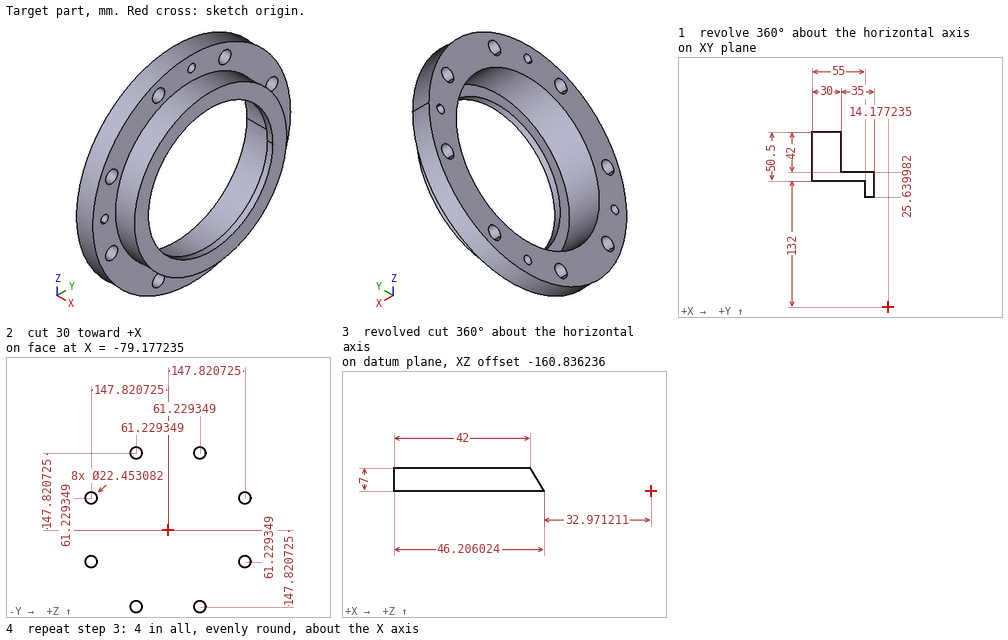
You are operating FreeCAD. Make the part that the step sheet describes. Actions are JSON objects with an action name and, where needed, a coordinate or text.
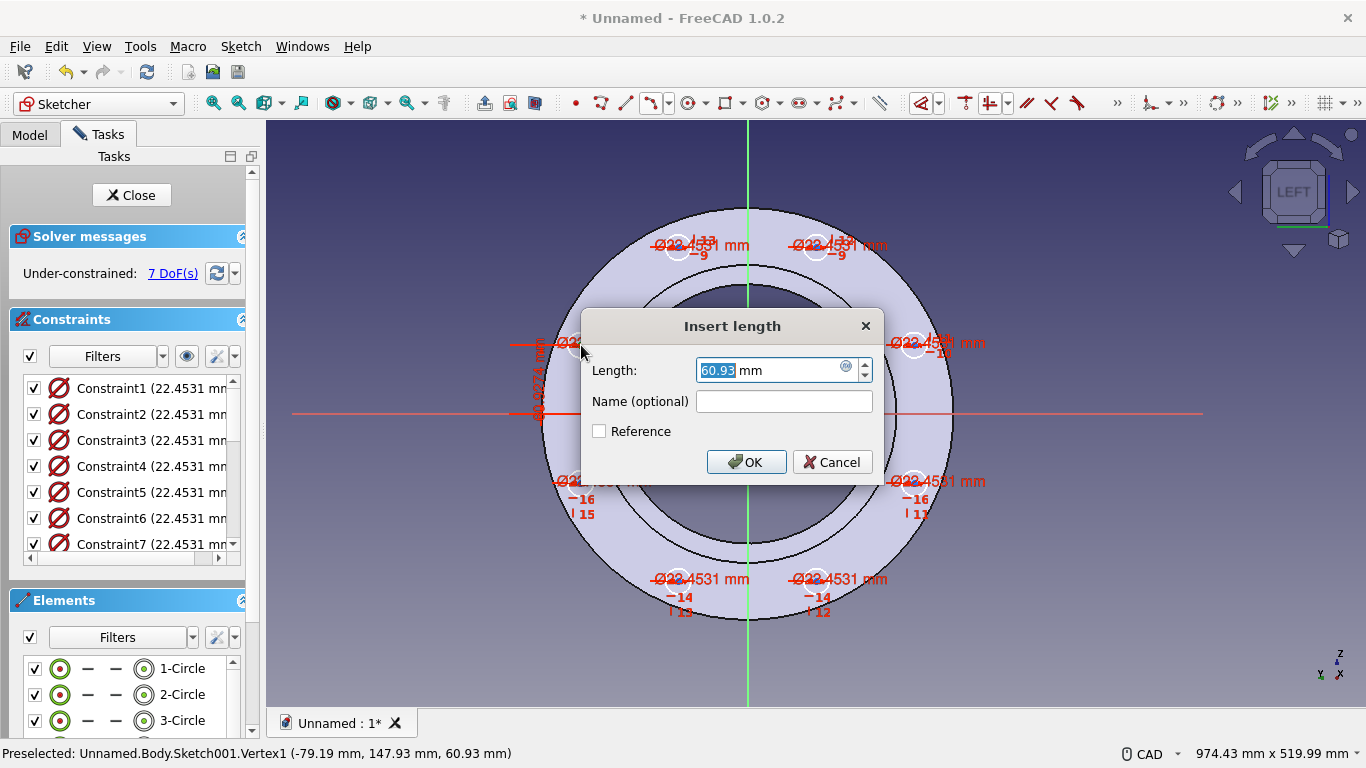
{"action": "type", "text": "61.229349"}
{"action": "key", "text": "Return"}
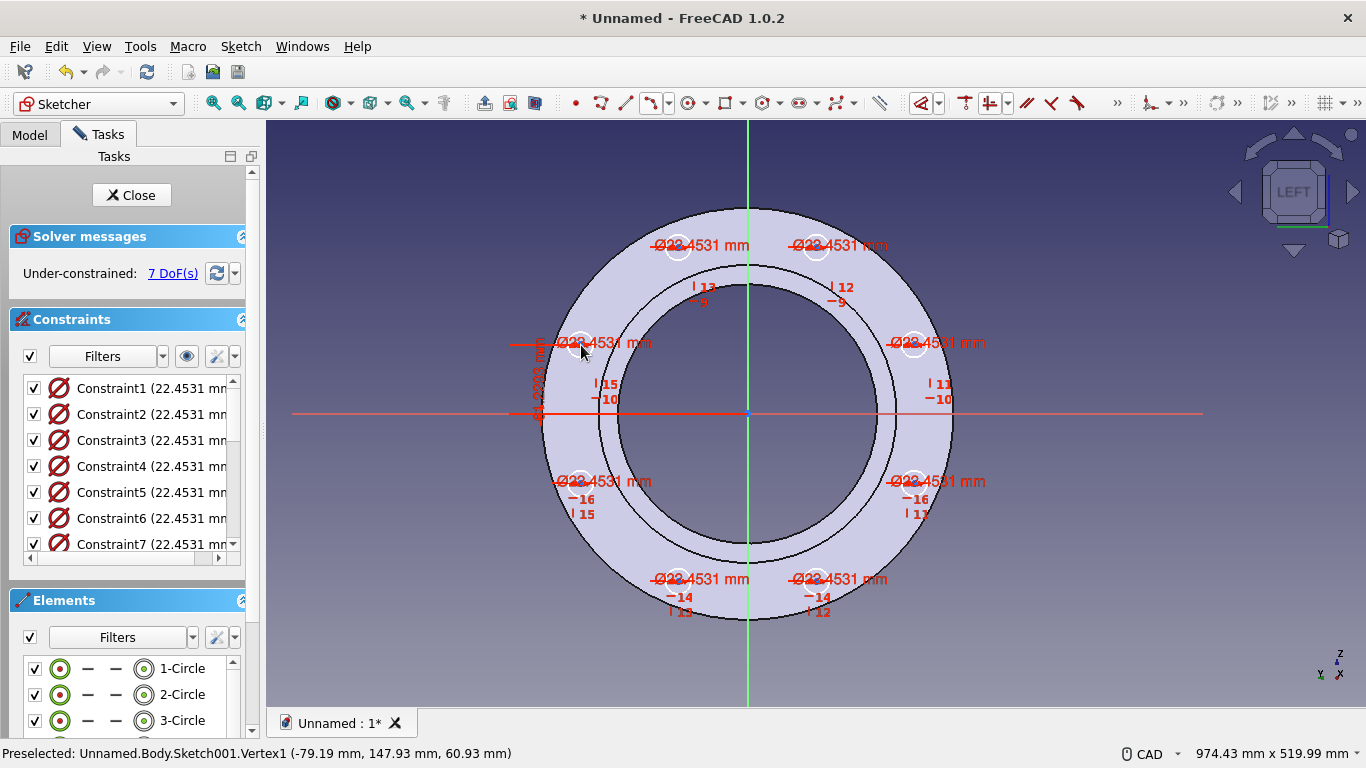
{"action": "left_click", "coordinate": [678, 247]}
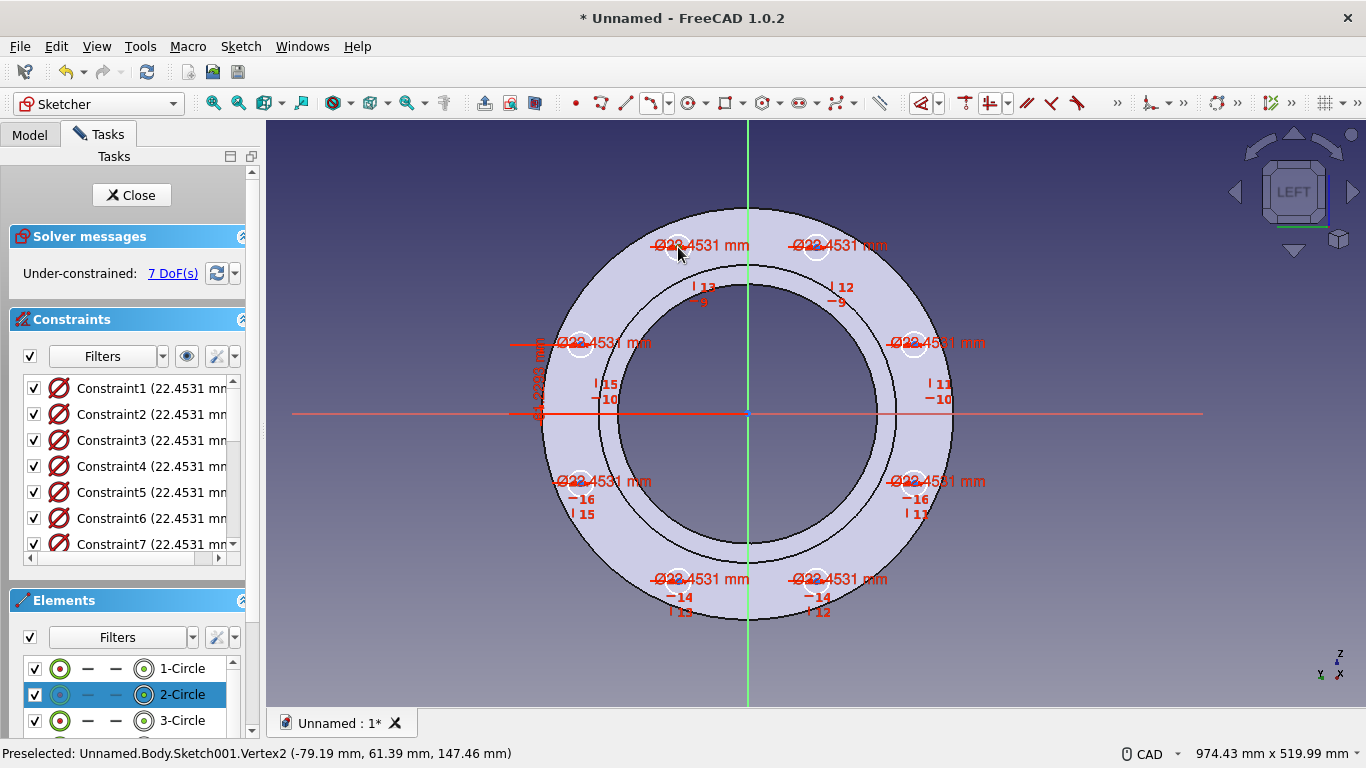
{"action": "left_click", "coordinate": [938, 104]}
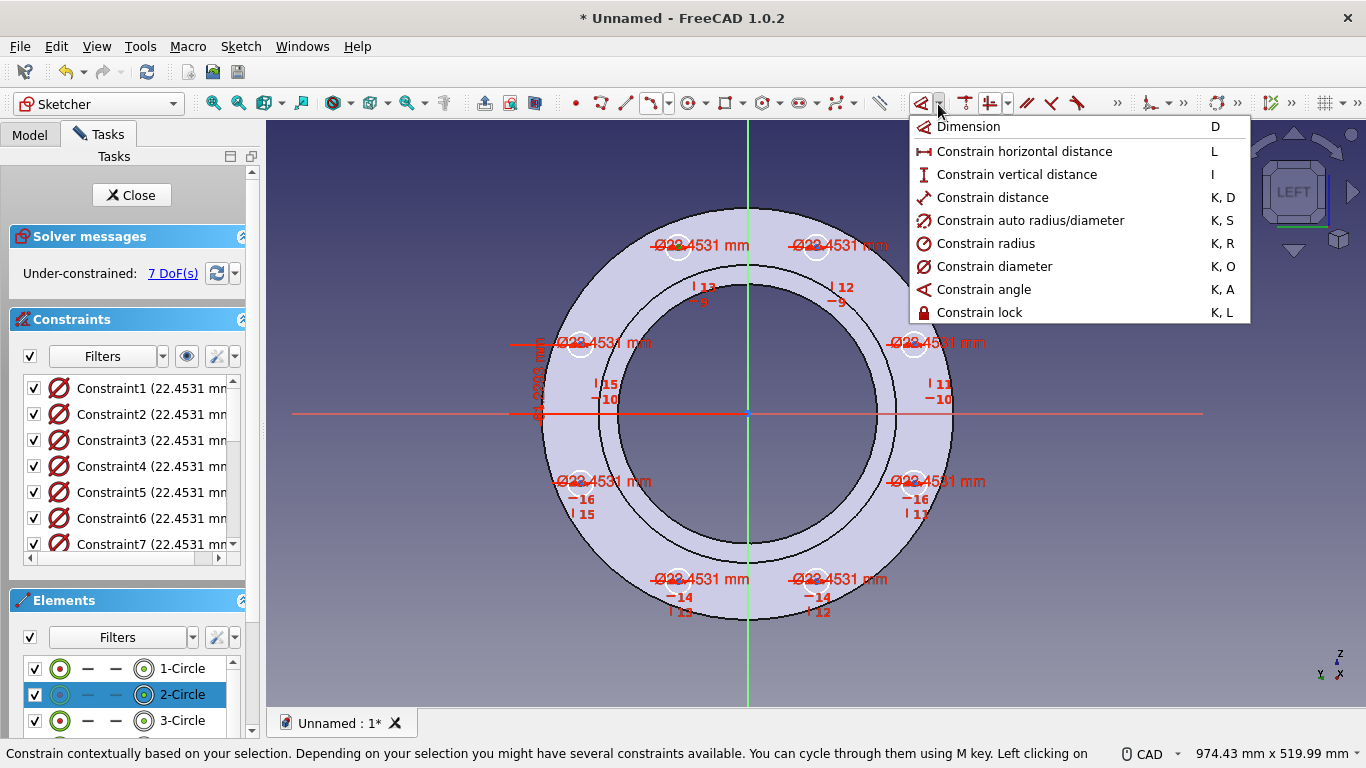
{"action": "left_click", "coordinate": [1080, 152]}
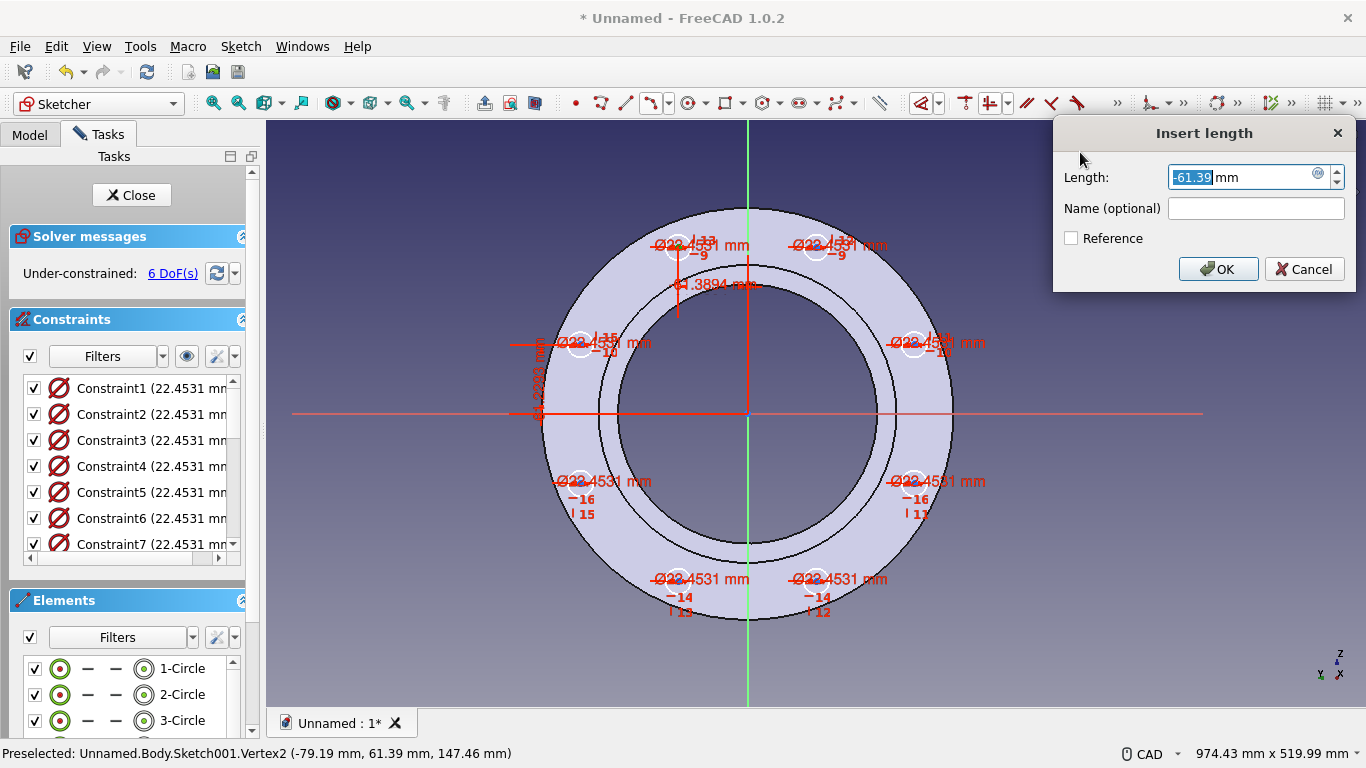
{"action": "type", "text": "-61.229349"}
{"action": "key", "text": "Return"}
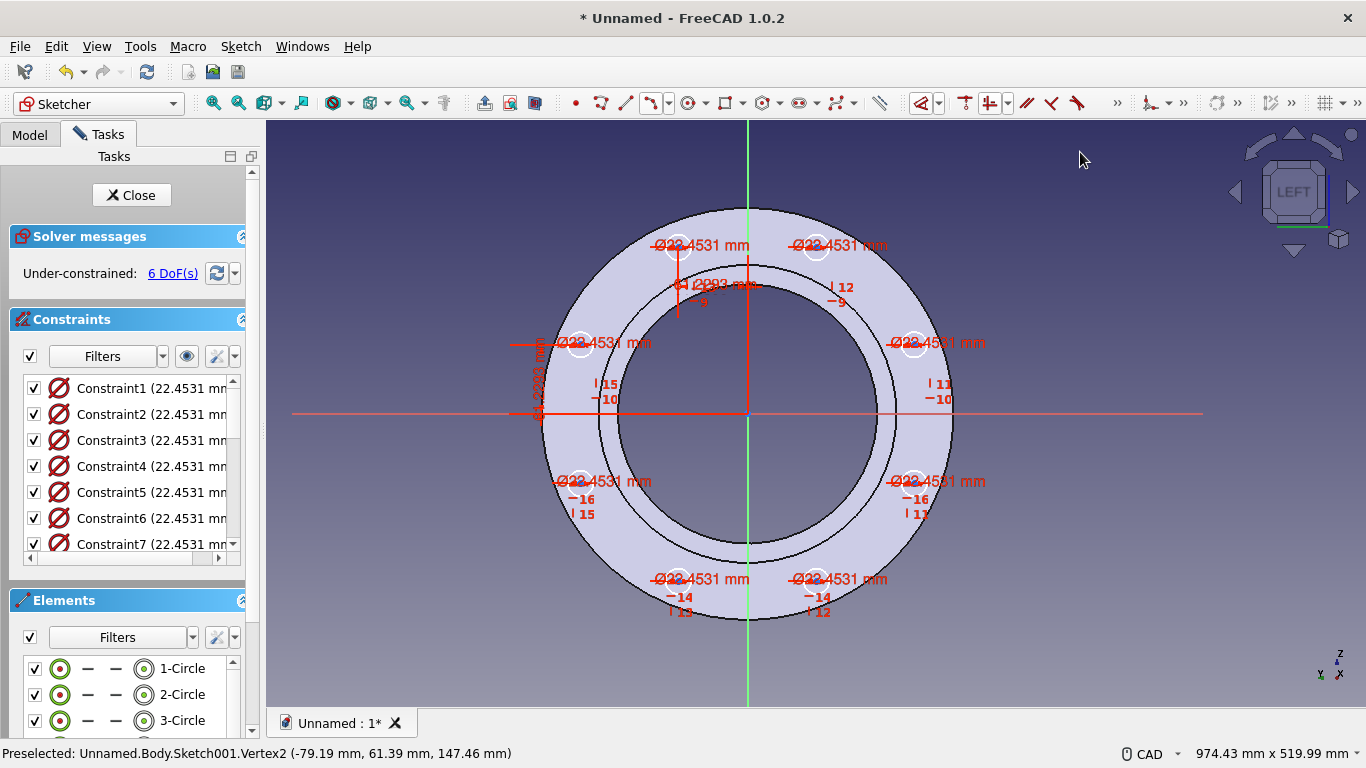
{"action": "left_click", "coordinate": [817, 247]}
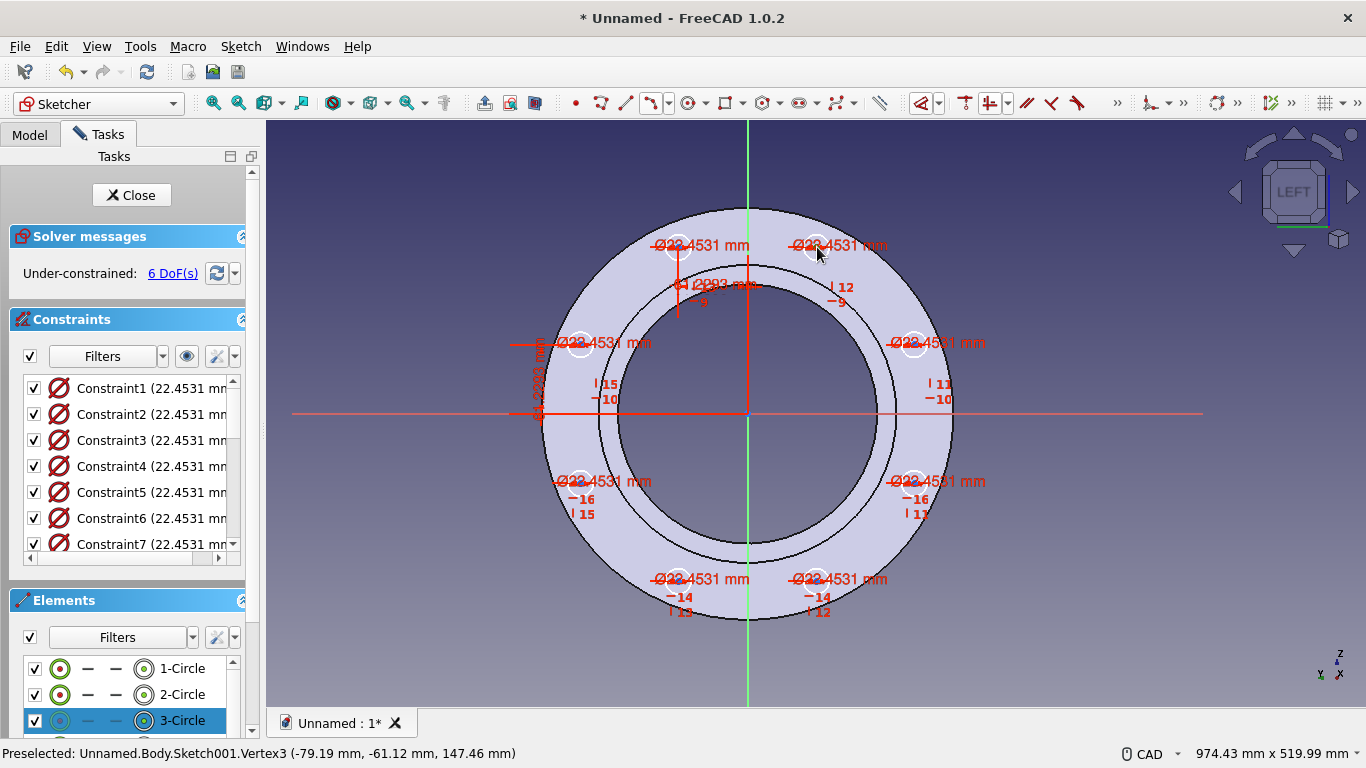
{"action": "left_click", "coordinate": [938, 104]}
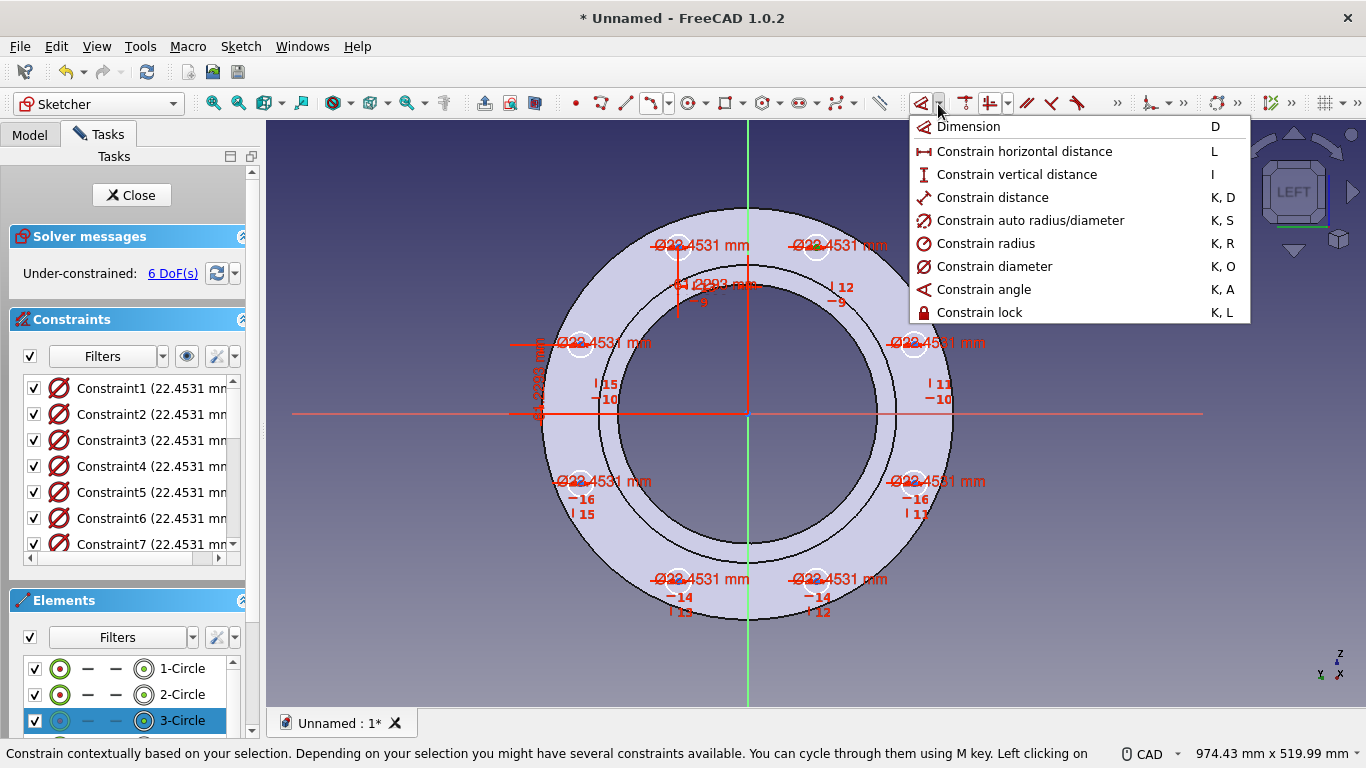
{"action": "left_click", "coordinate": [1080, 152]}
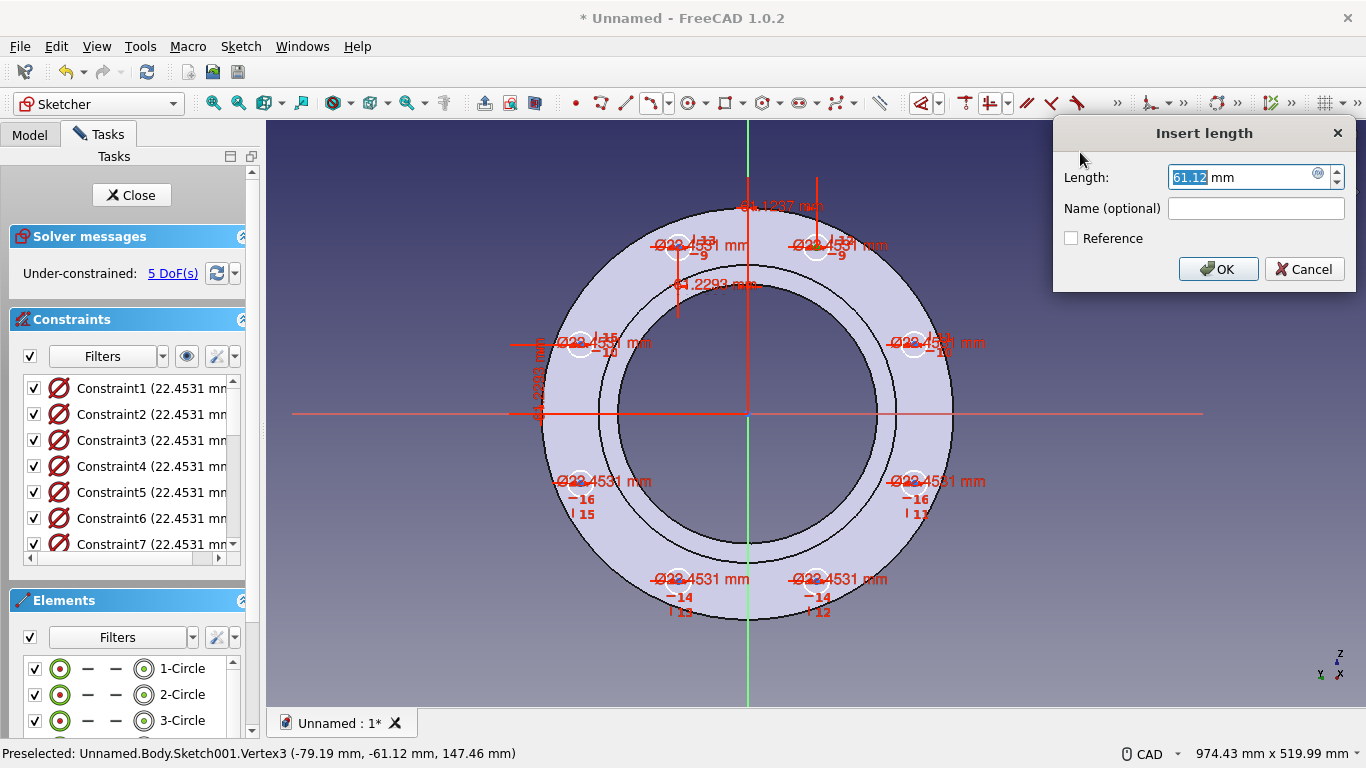
{"action": "type", "text": "61.229349"}
{"action": "key", "text": "Return"}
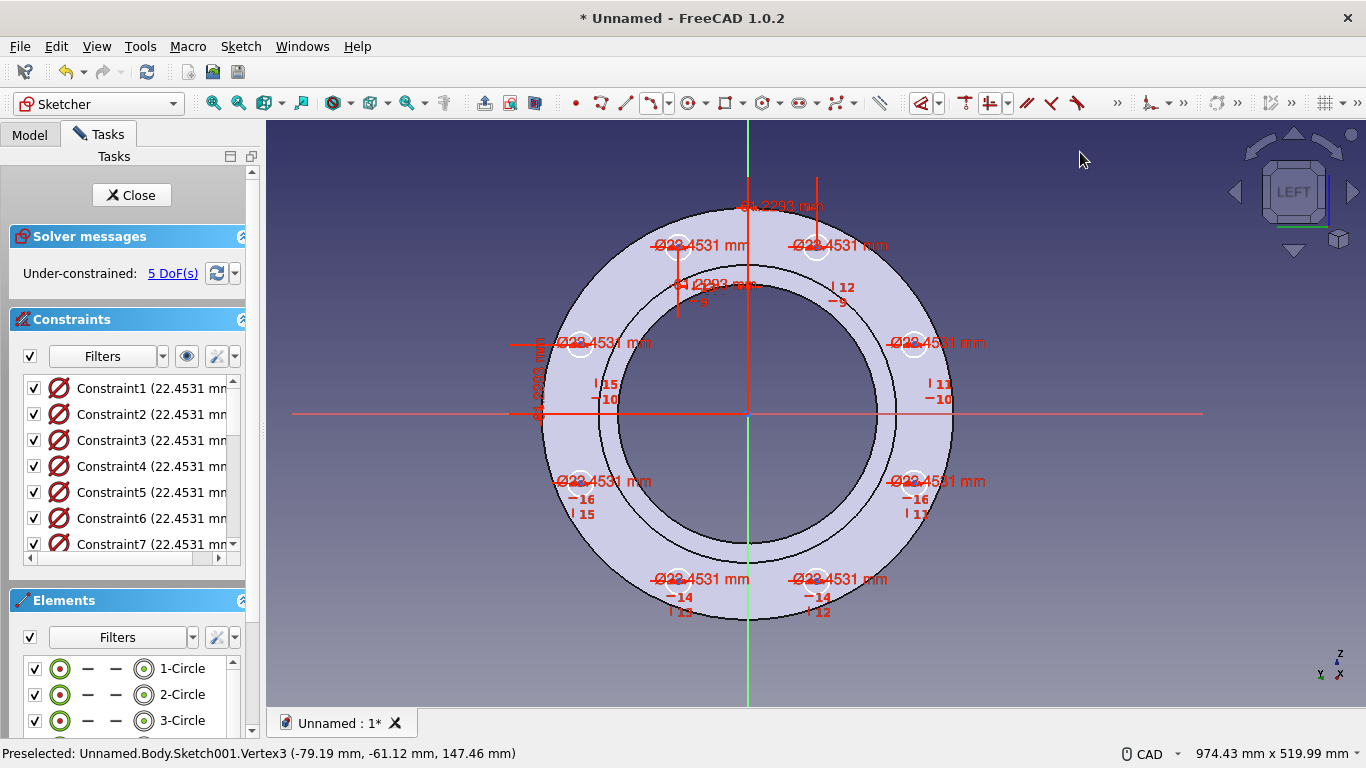
{"action": "left_click", "coordinate": [914, 483]}